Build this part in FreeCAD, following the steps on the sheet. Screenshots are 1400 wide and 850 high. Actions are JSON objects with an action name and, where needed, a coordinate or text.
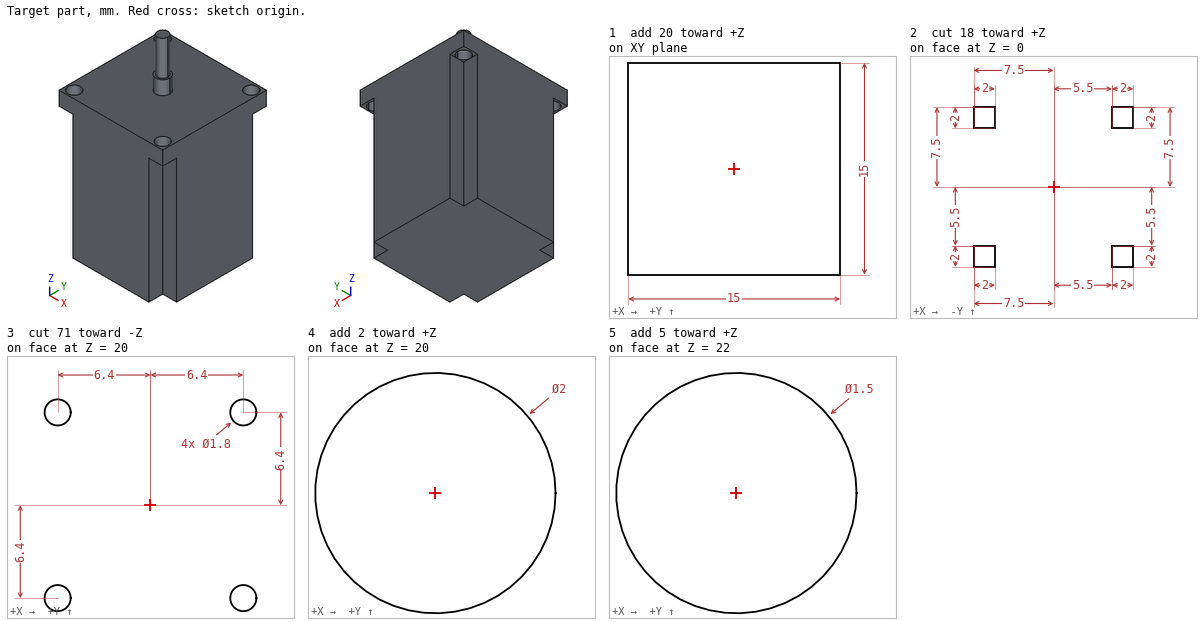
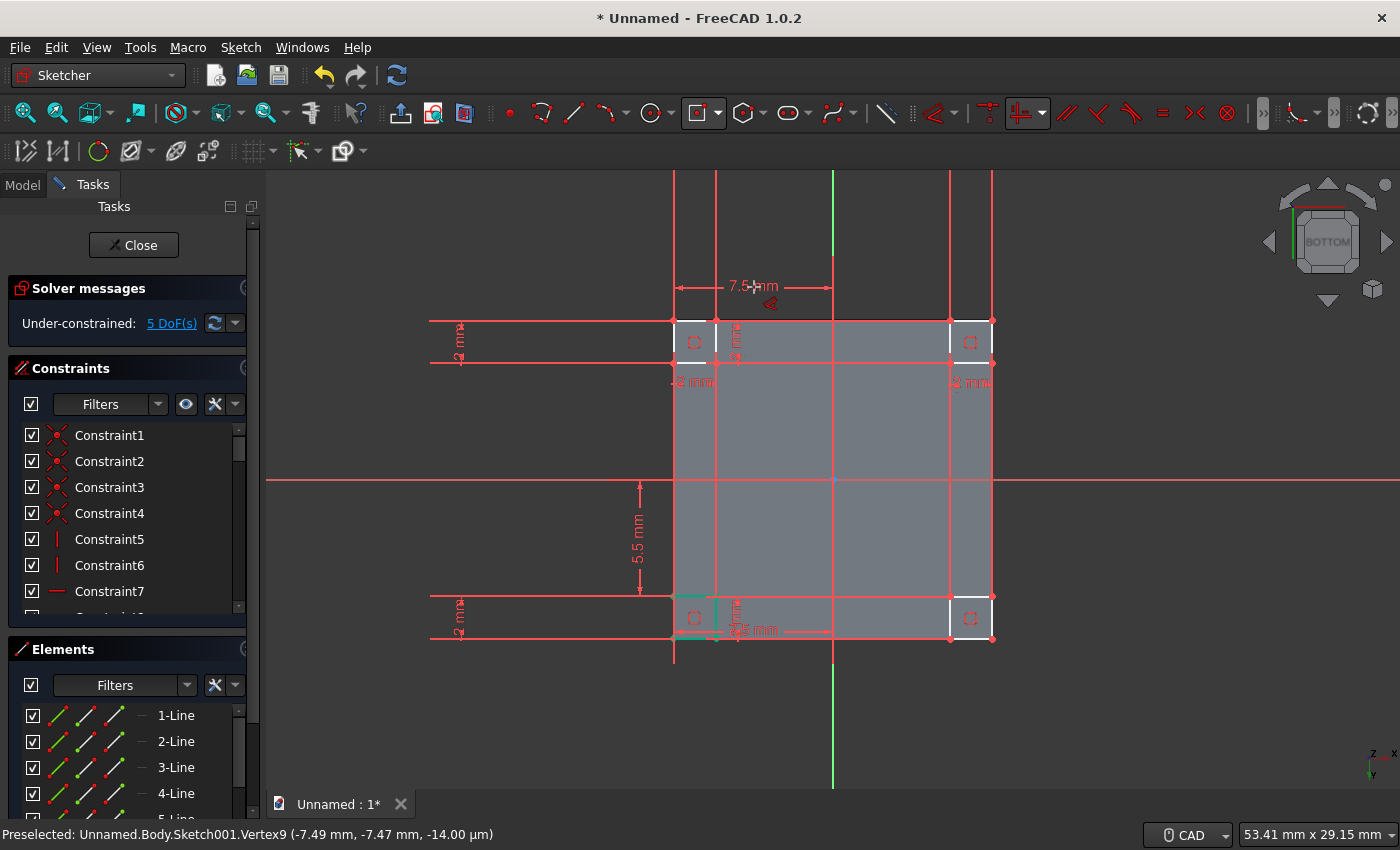
{"action": "left_click", "coordinate": [674, 321]}
{"action": "left_click", "coordinate": [640, 400]}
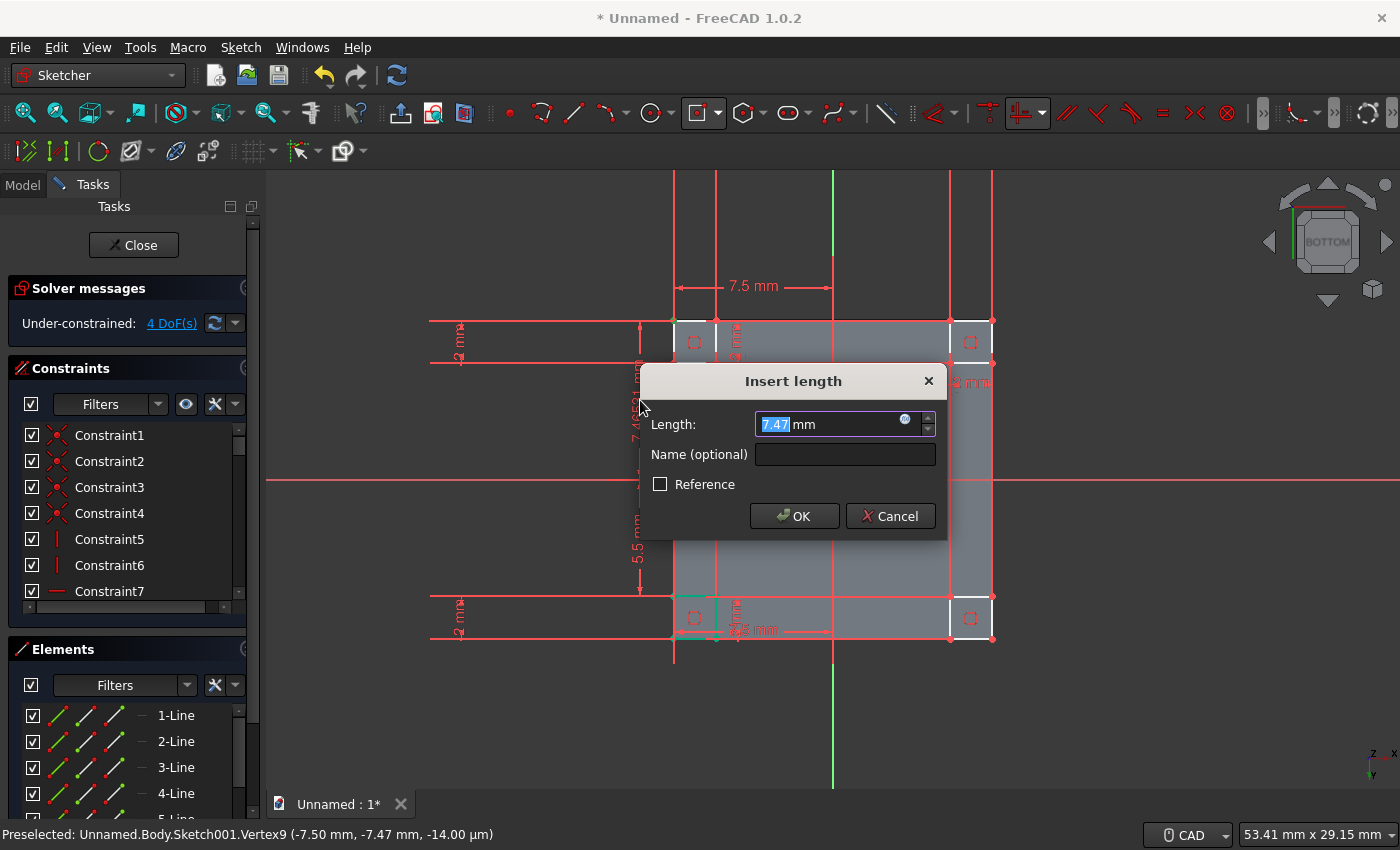
{"action": "type", "text": "7.5"}
{"action": "key", "text": "Return"}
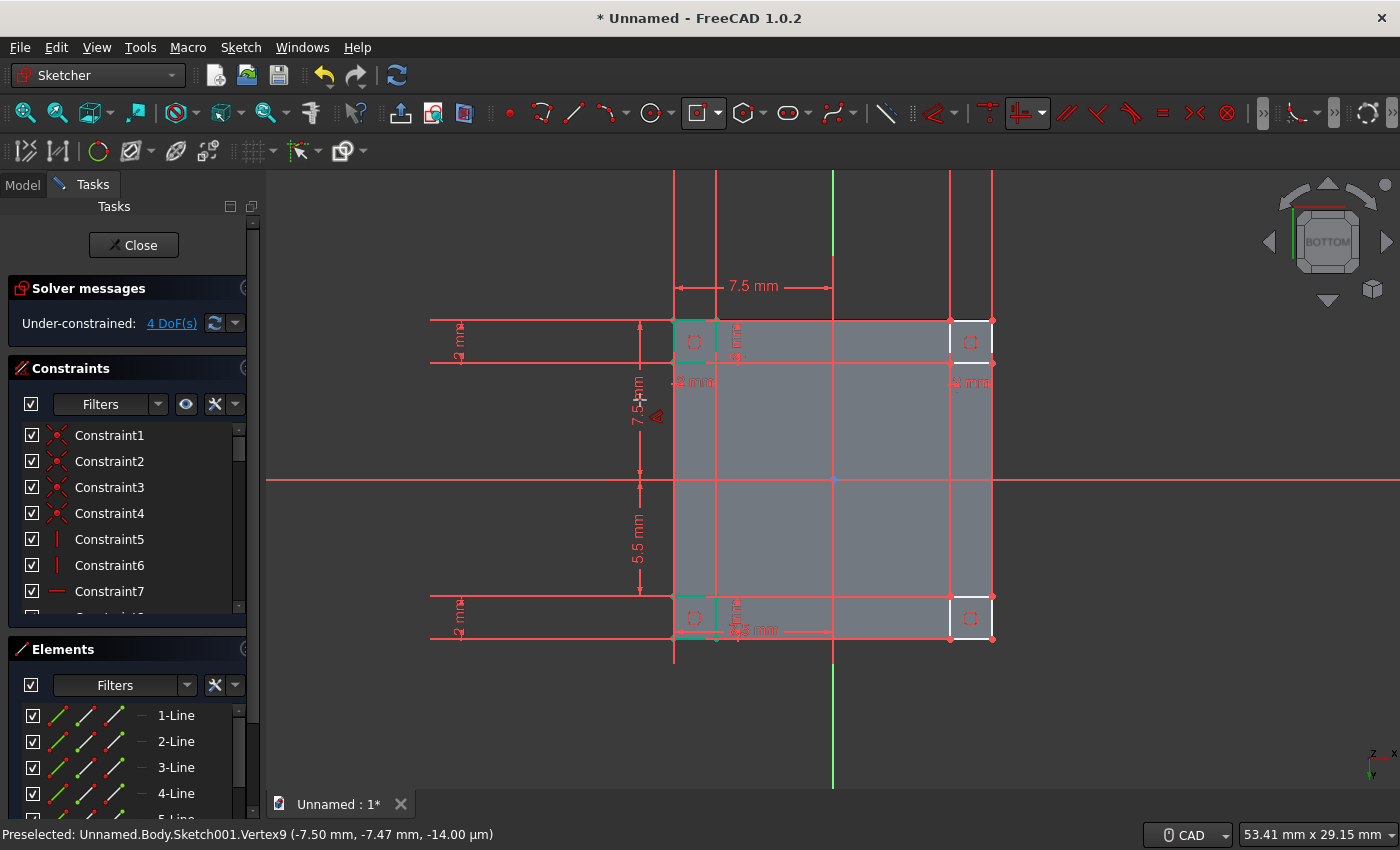
{"action": "left_click", "coordinate": [950, 321]}
{"action": "left_click", "coordinate": [892, 287]}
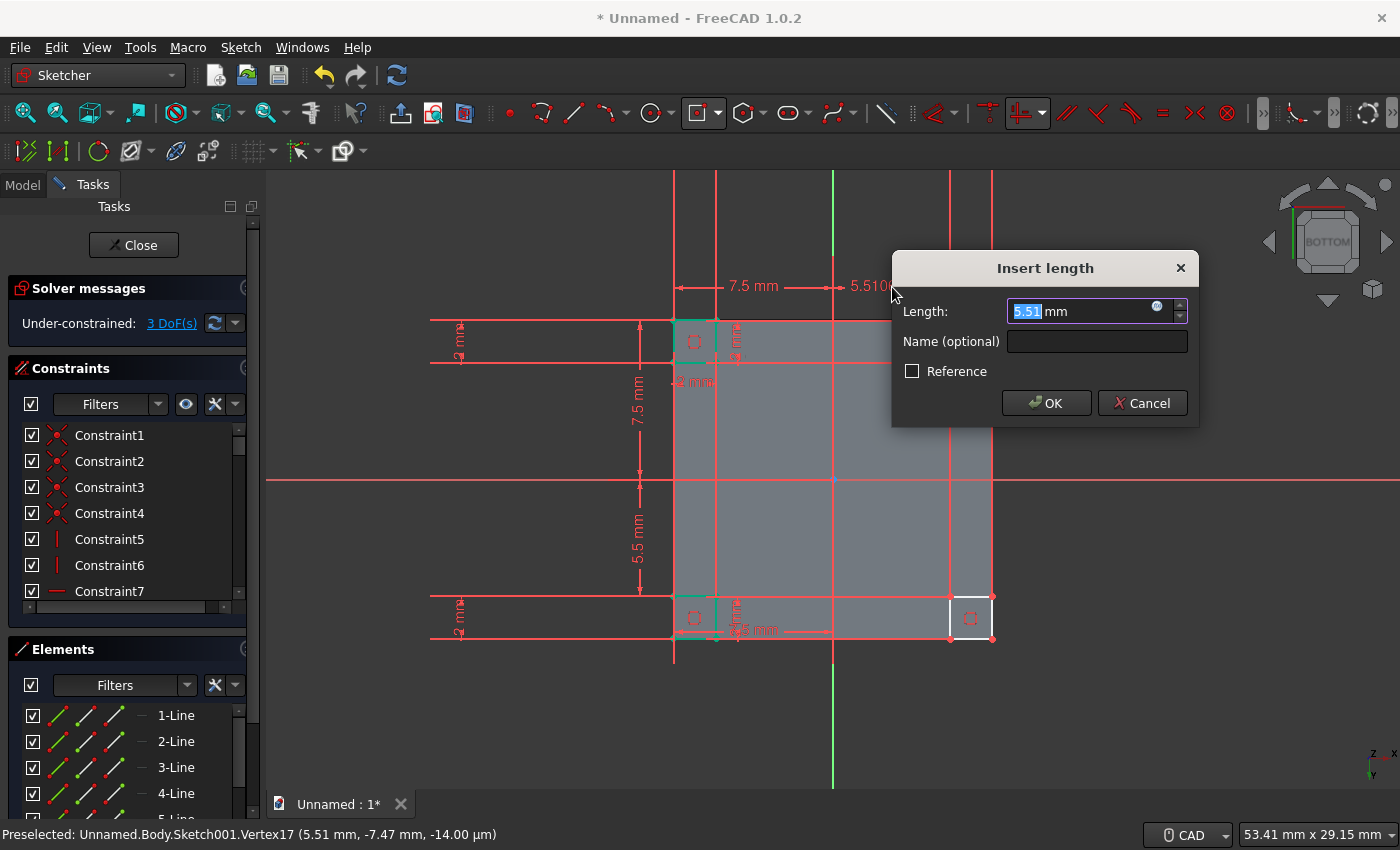
{"action": "type", "text": "5.5"}
{"action": "key", "text": "Return"}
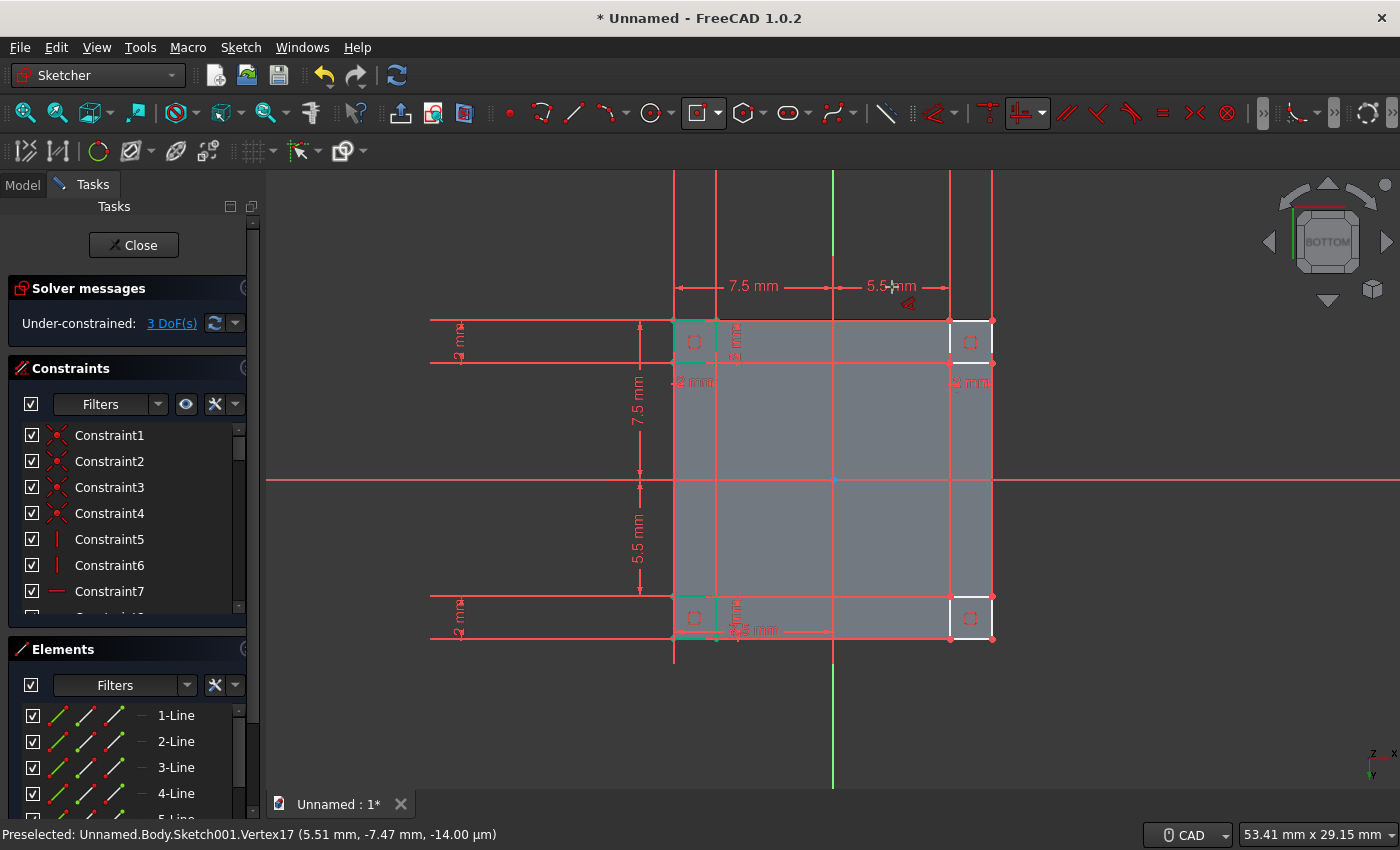
{"action": "left_click", "coordinate": [950, 321]}
{"action": "left_click", "coordinate": [984, 400]}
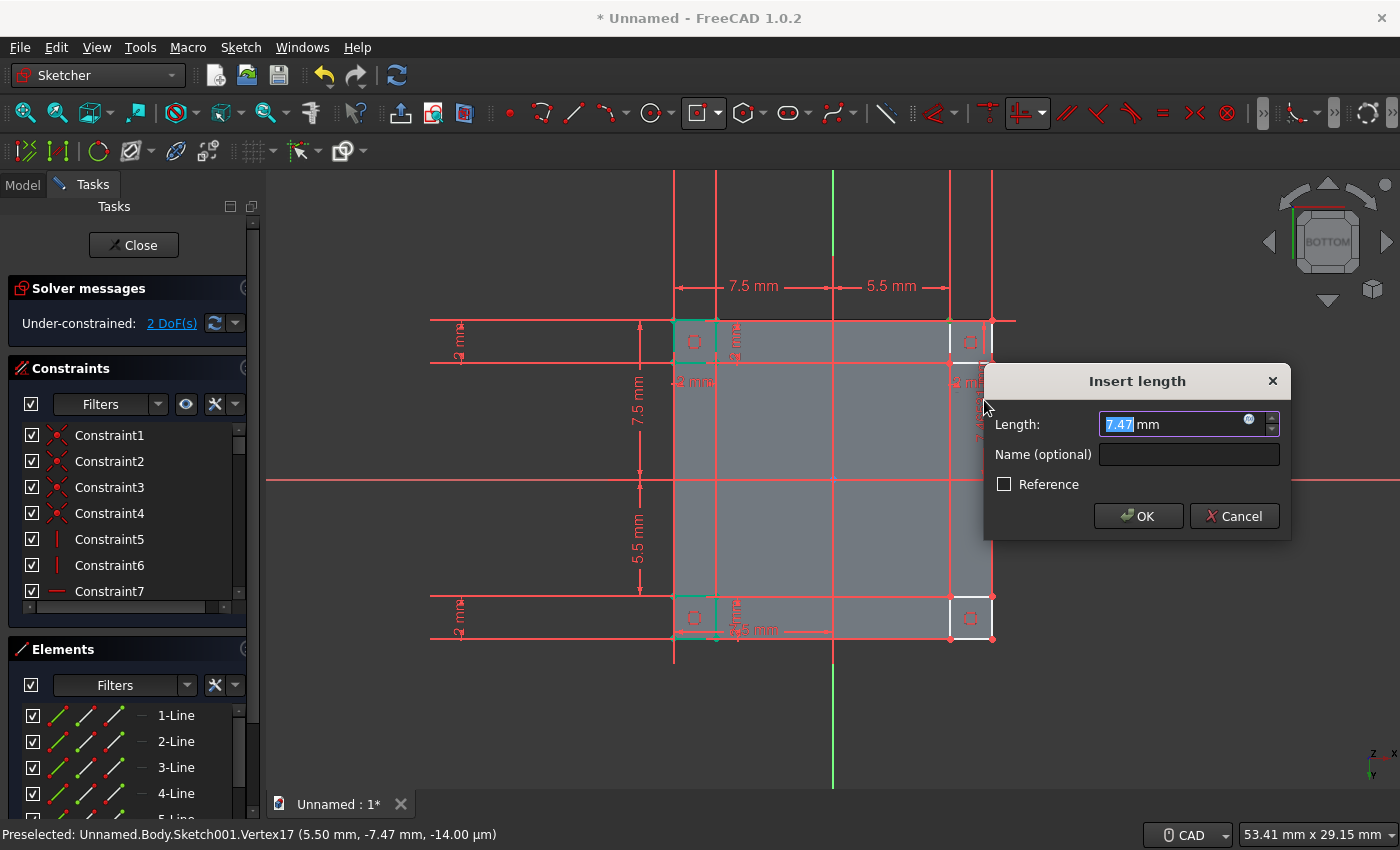
{"action": "type", "text": "7.5"}
{"action": "key", "text": "Return"}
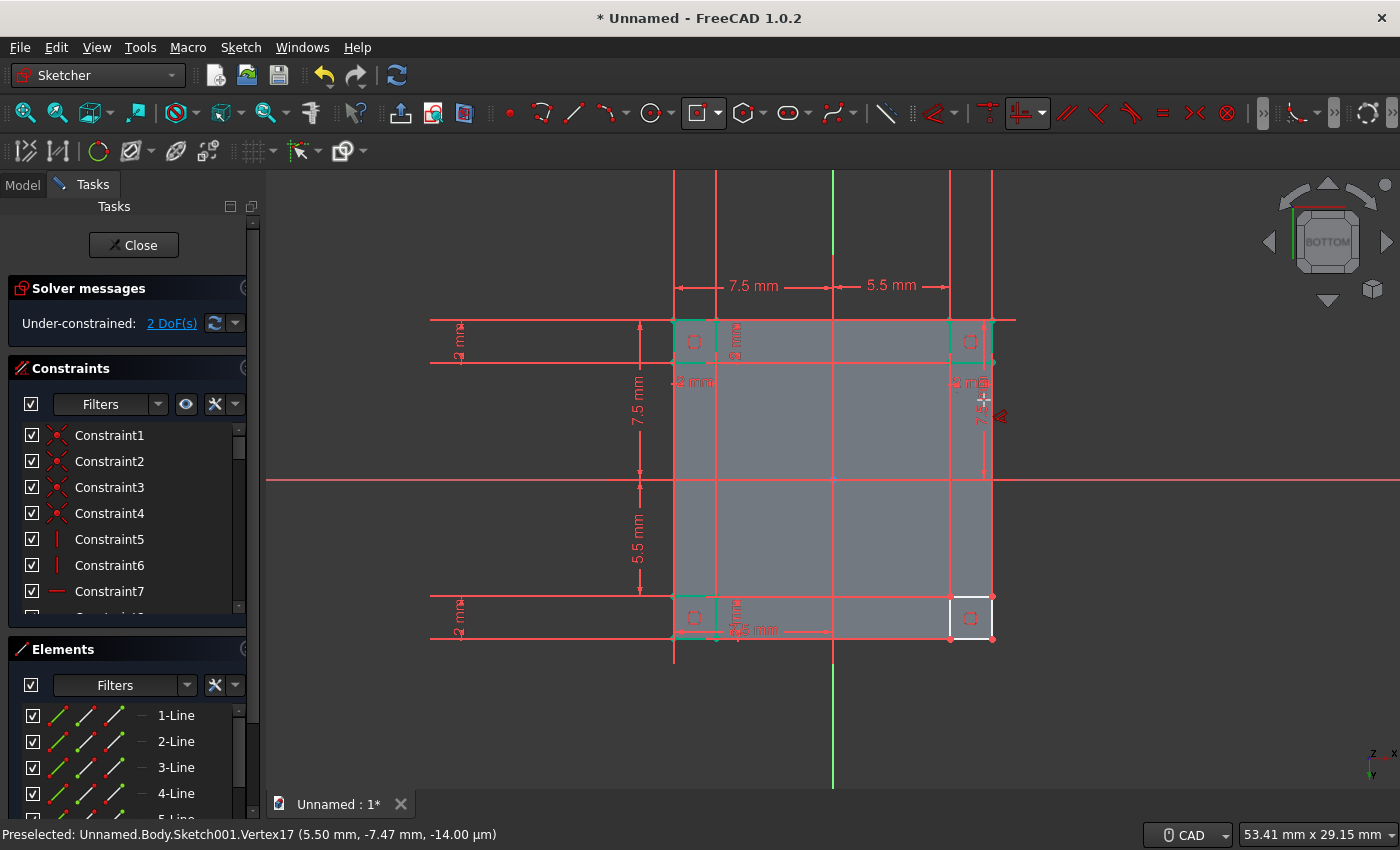
{"action": "left_click", "coordinate": [950, 597]}
{"action": "left_click", "coordinate": [892, 631]}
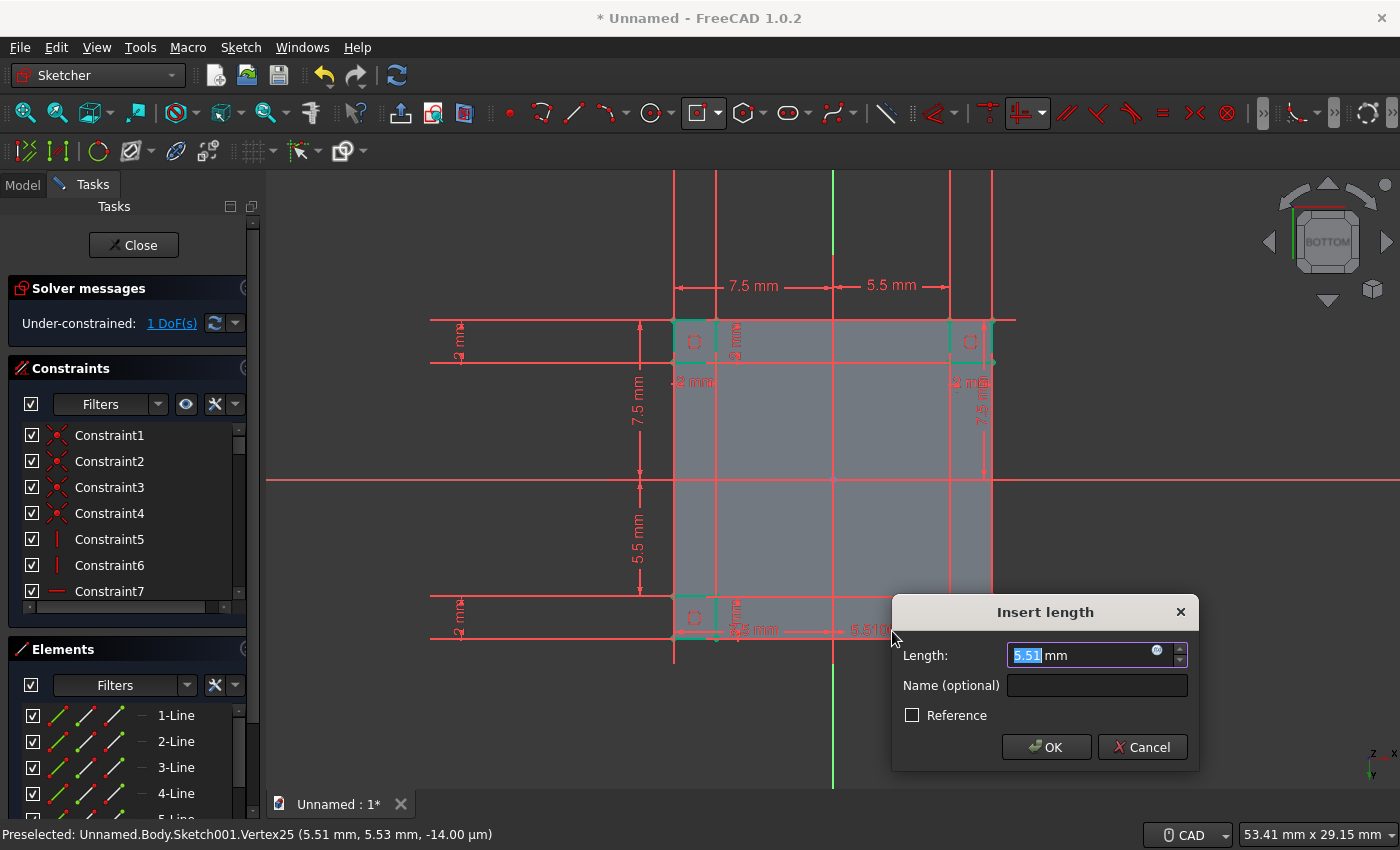
{"action": "type", "text": "5.5"}
{"action": "key", "text": "Return"}